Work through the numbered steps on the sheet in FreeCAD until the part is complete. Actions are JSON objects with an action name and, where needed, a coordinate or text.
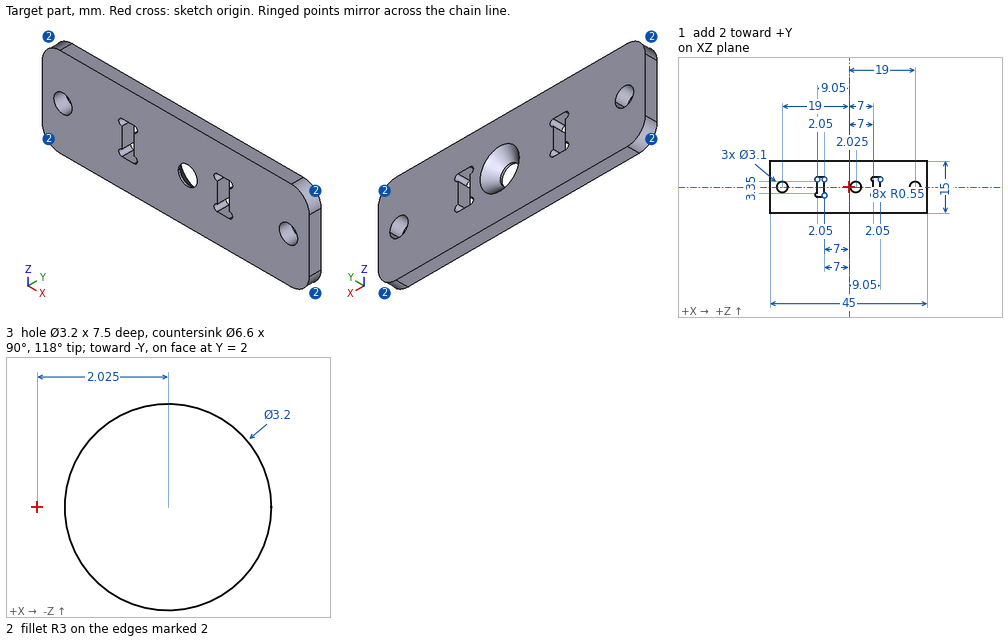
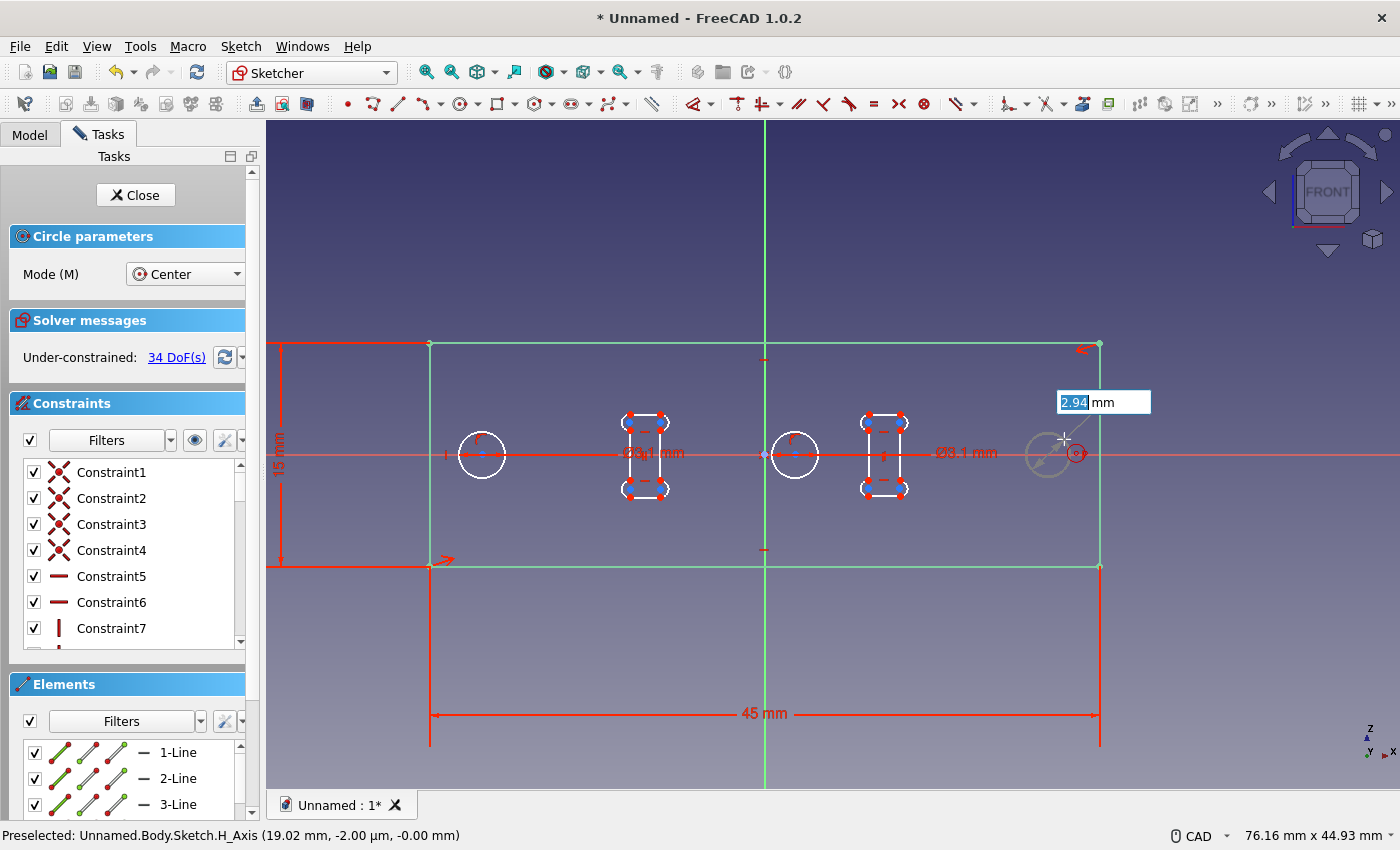
{"action": "type", "text": "3.1"}
{"action": "key", "text": "Return"}
{"action": "key", "text": "Escape"}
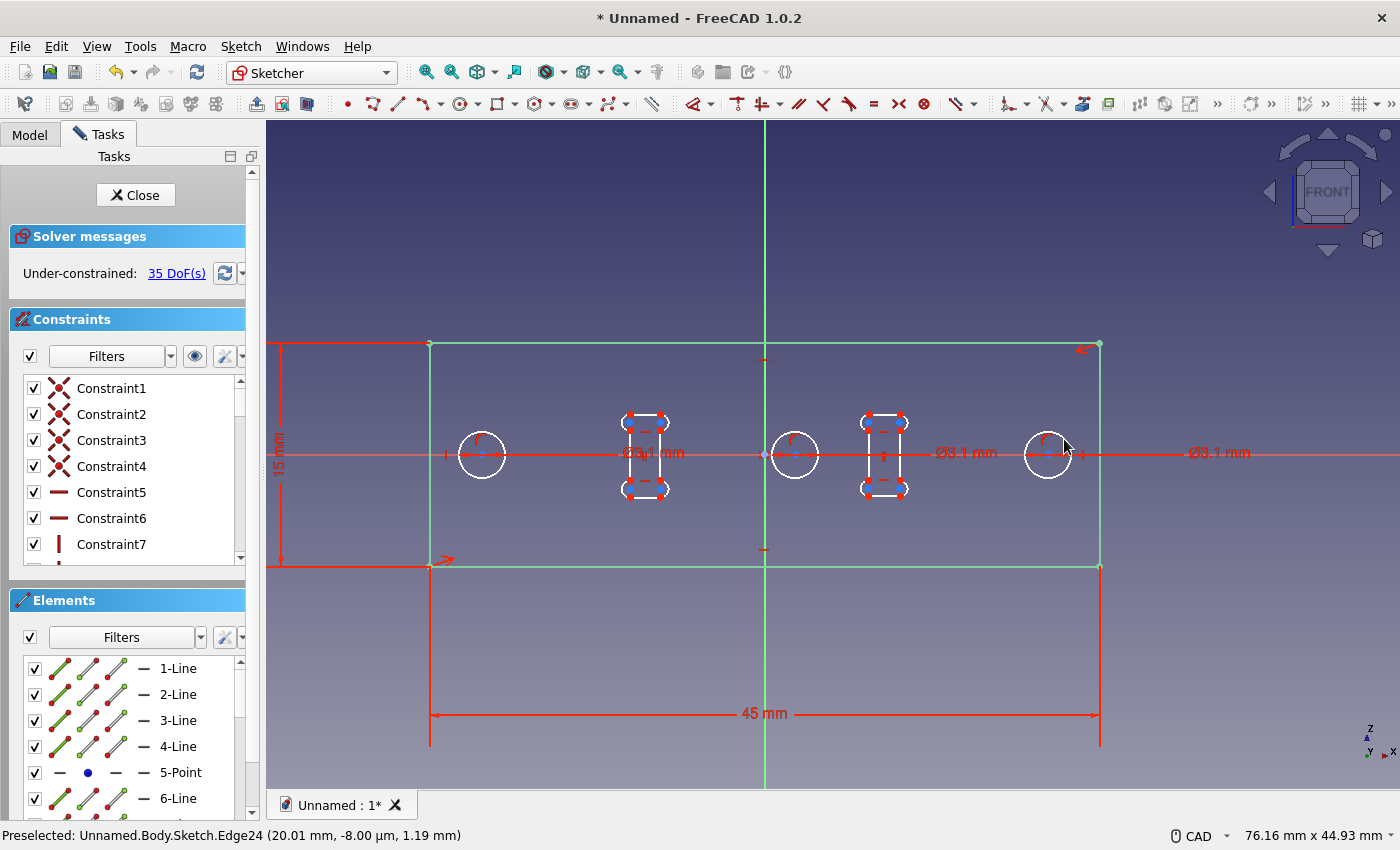
{"action": "left_click", "coordinate": [642, 498]}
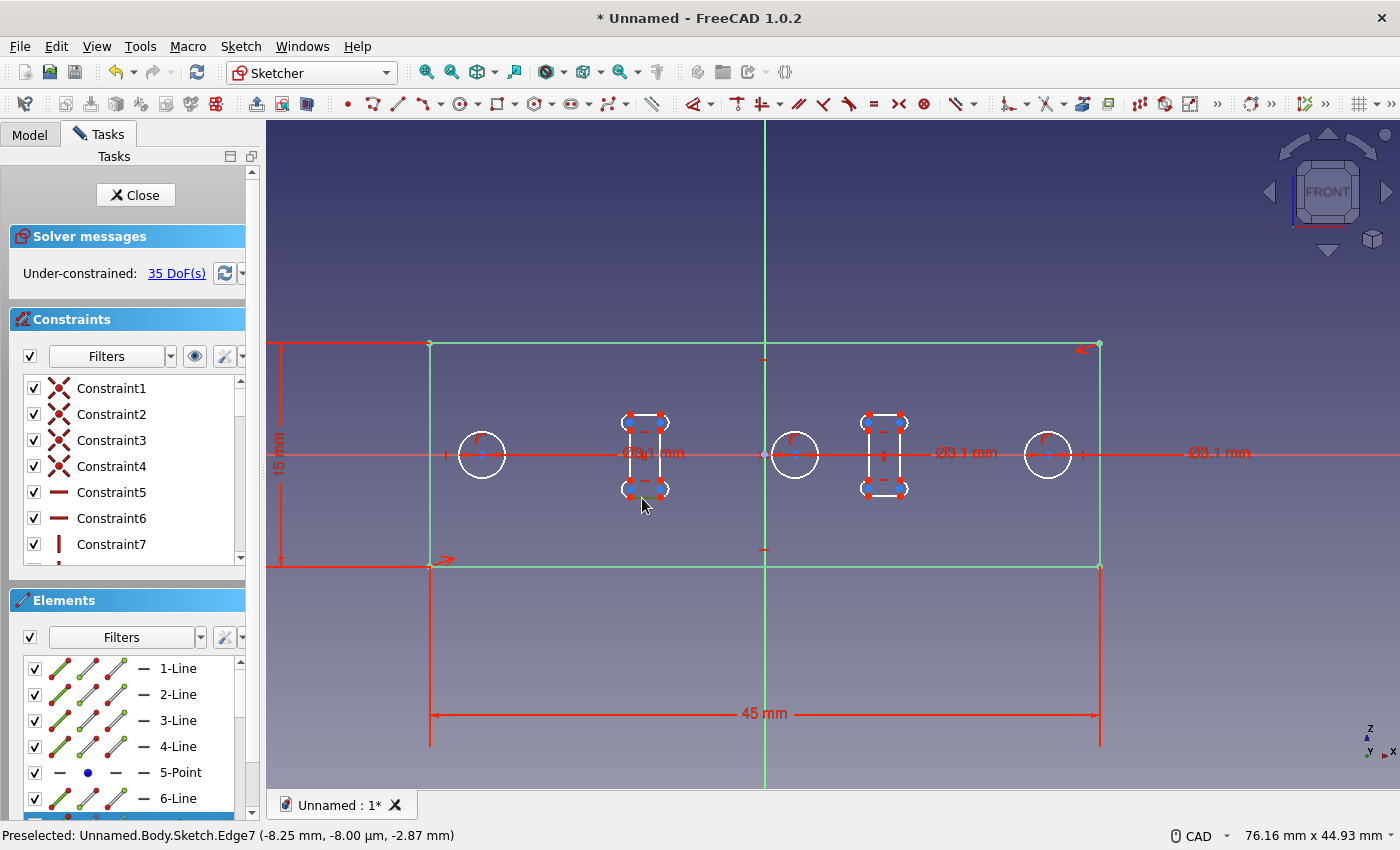
{"action": "scroll", "coordinate": [622, 489], "scroll_direction": "up", "scroll_amount": 3}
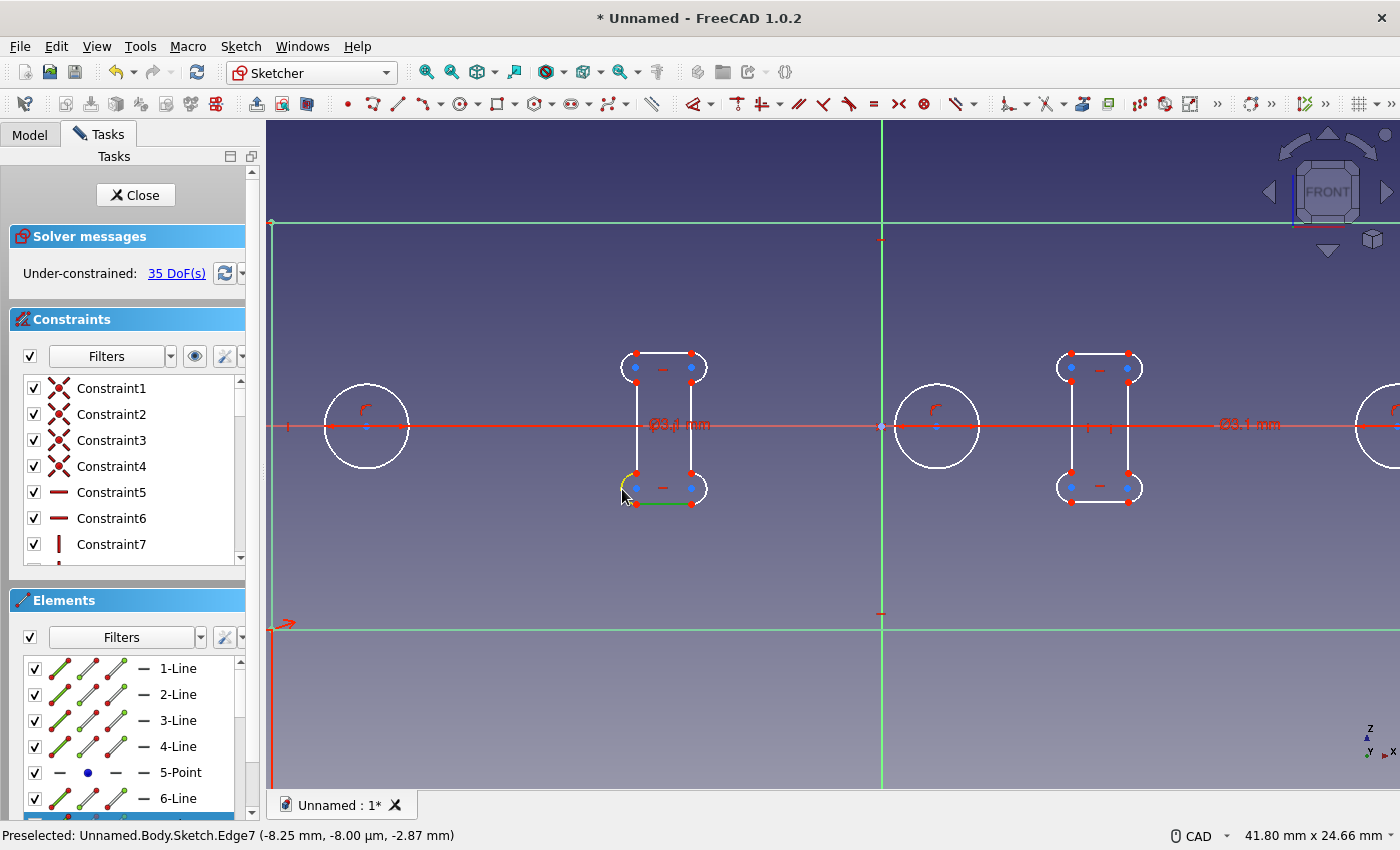
{"action": "left_click", "coordinate": [621, 489]}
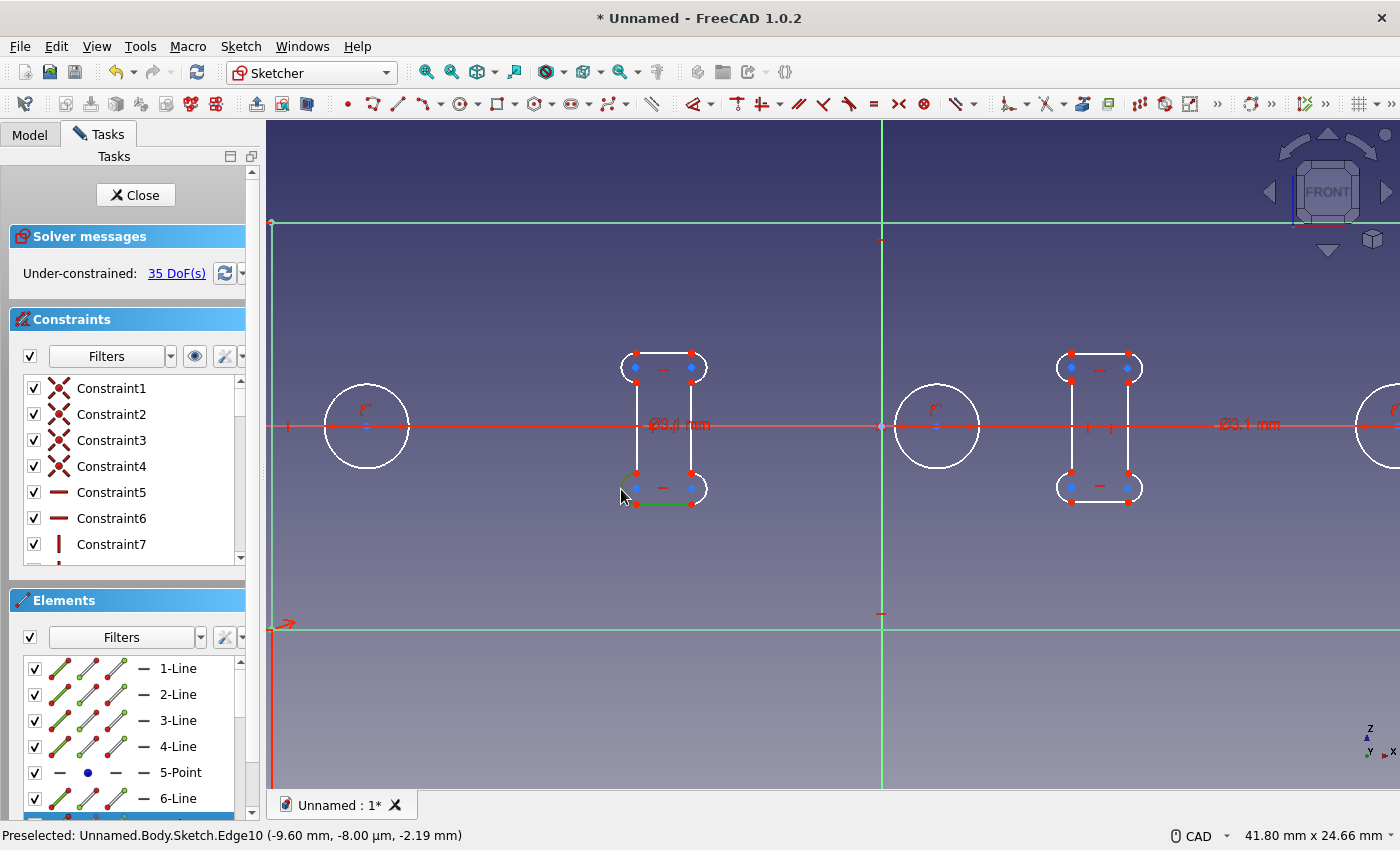
{"action": "left_click", "coordinate": [849, 104]}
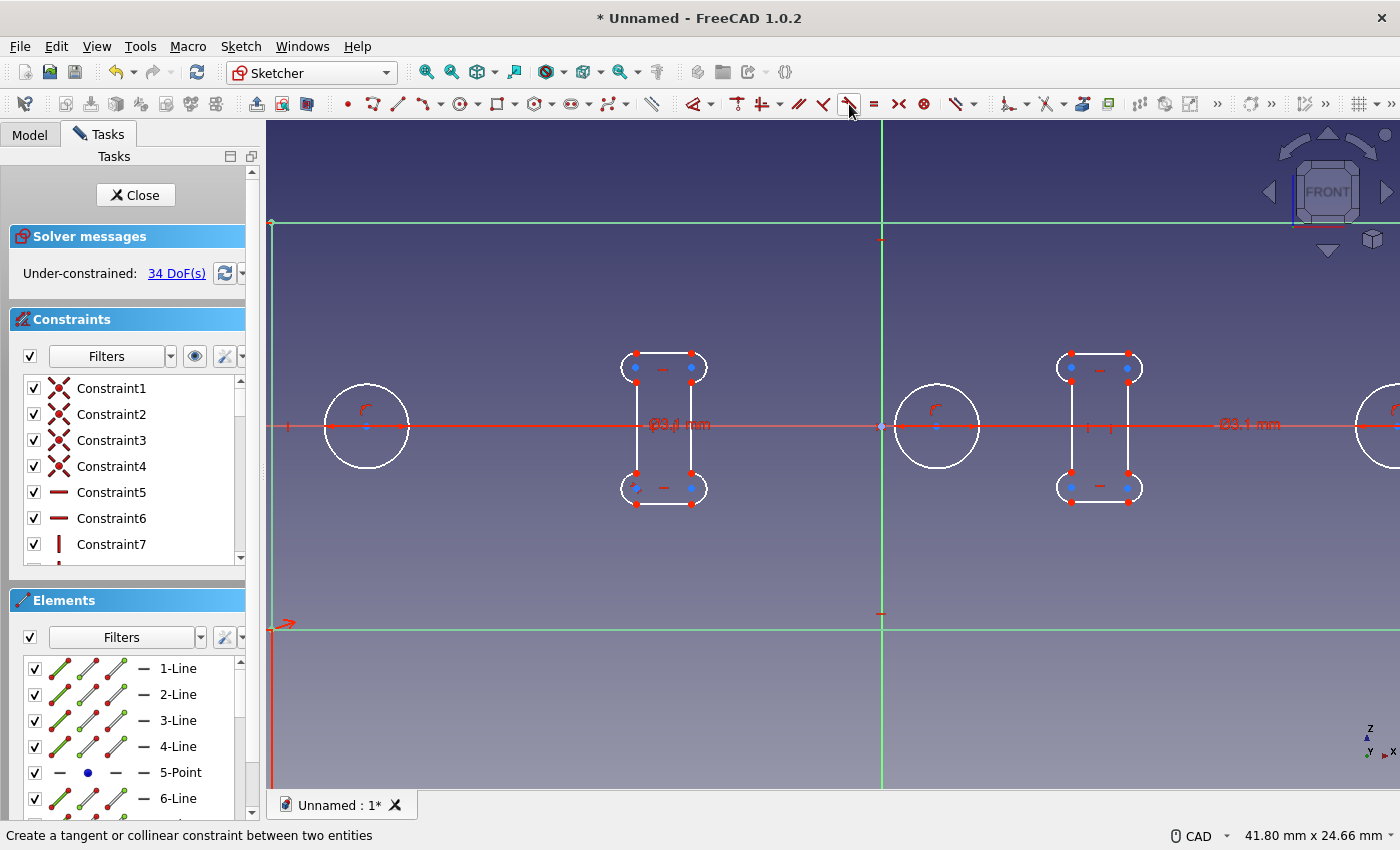
{"action": "left_click", "coordinate": [653, 504]}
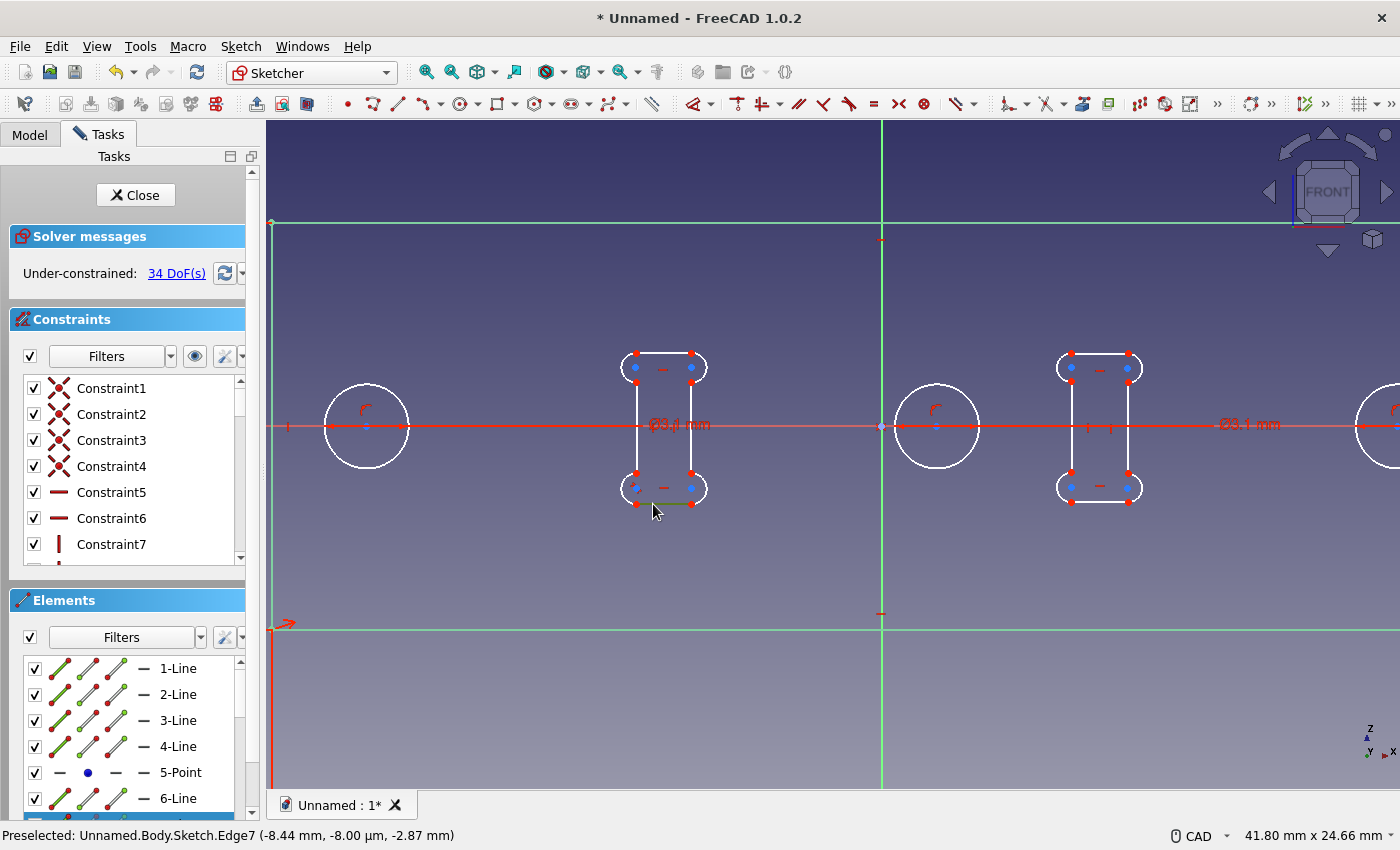
{"action": "left_click", "coordinate": [704, 498]}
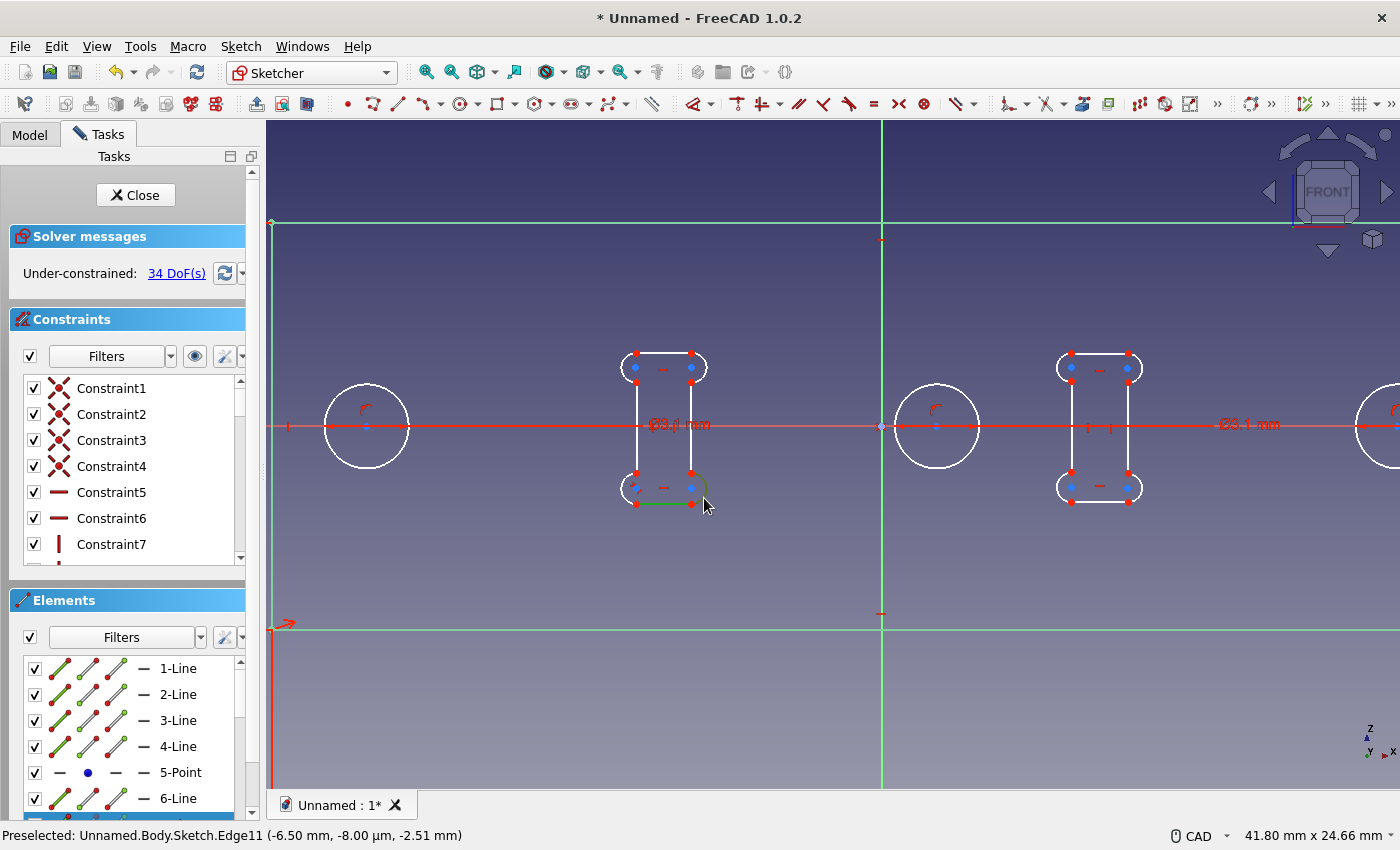
{"action": "left_click", "coordinate": [849, 104]}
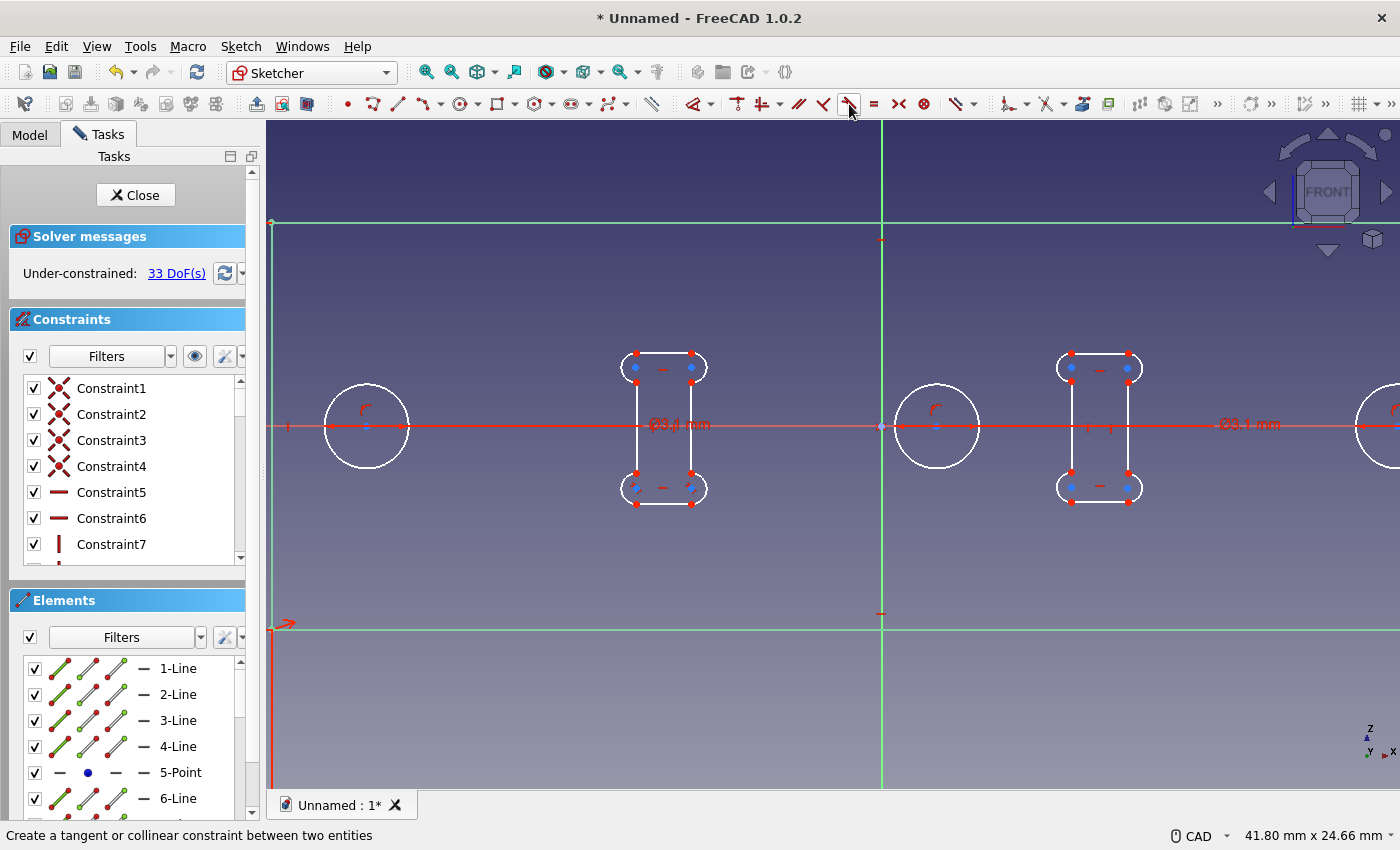
{"action": "left_click", "coordinate": [675, 353]}